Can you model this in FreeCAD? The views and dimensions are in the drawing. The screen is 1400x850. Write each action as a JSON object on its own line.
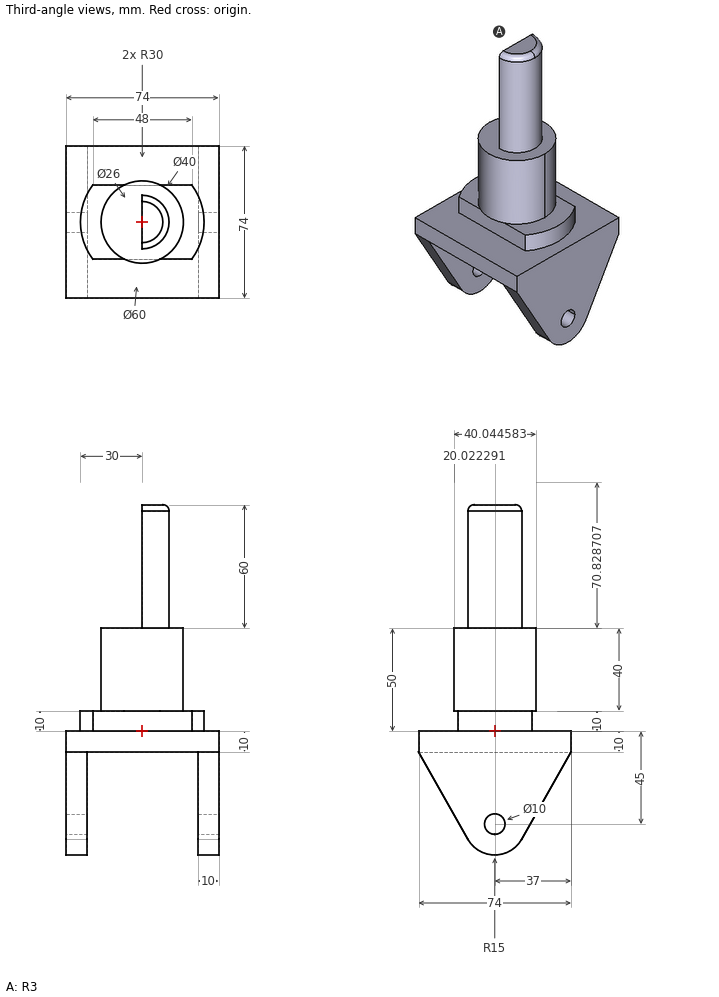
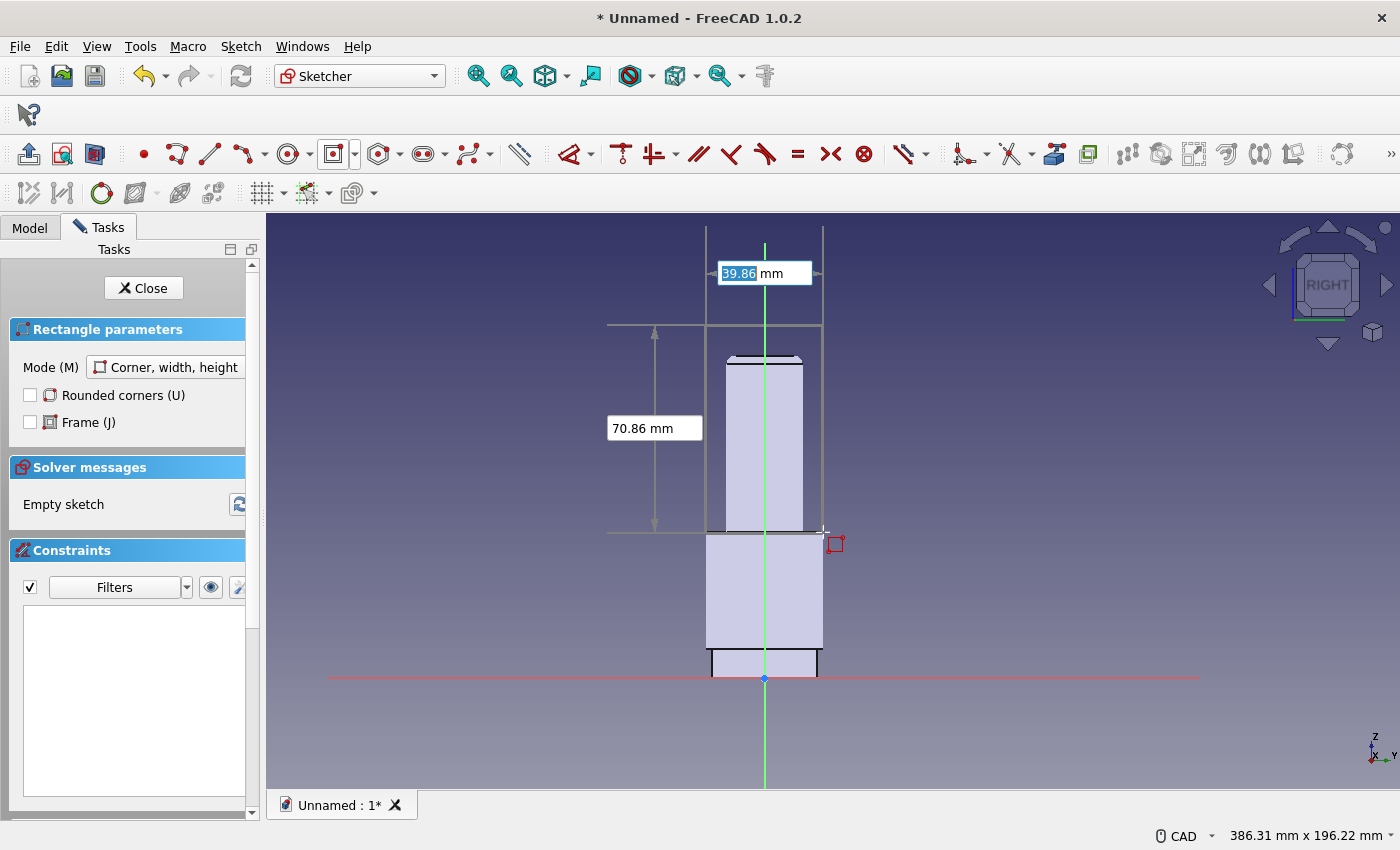
{"action": "type", "text": "40.044583"}
{"action": "key", "text": "Tab"}
{"action": "type", "text": "70.828707"}
{"action": "key", "text": "Return"}
{"action": "key", "text": "Escape"}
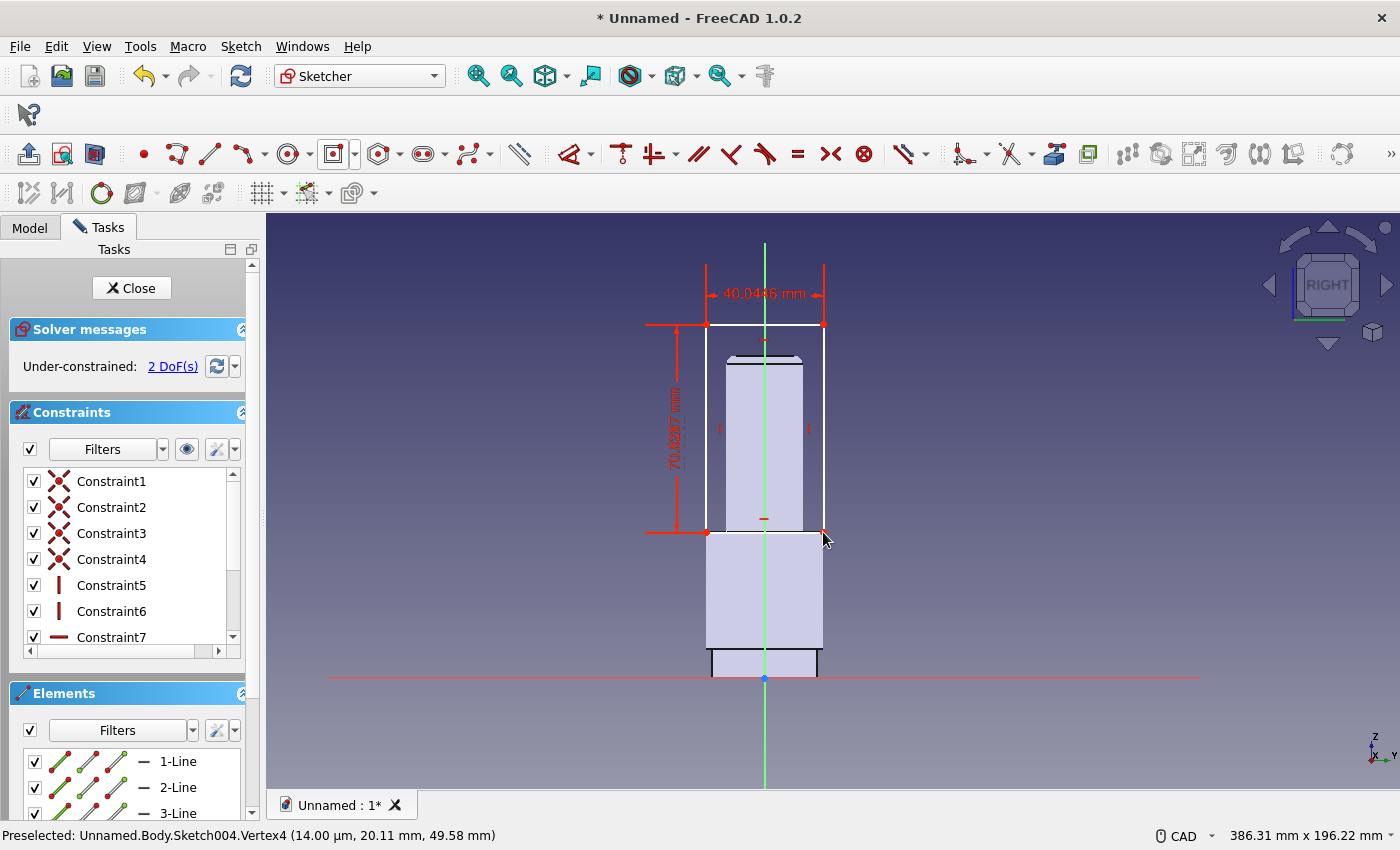
{"action": "left_click", "coordinate": [568, 154]}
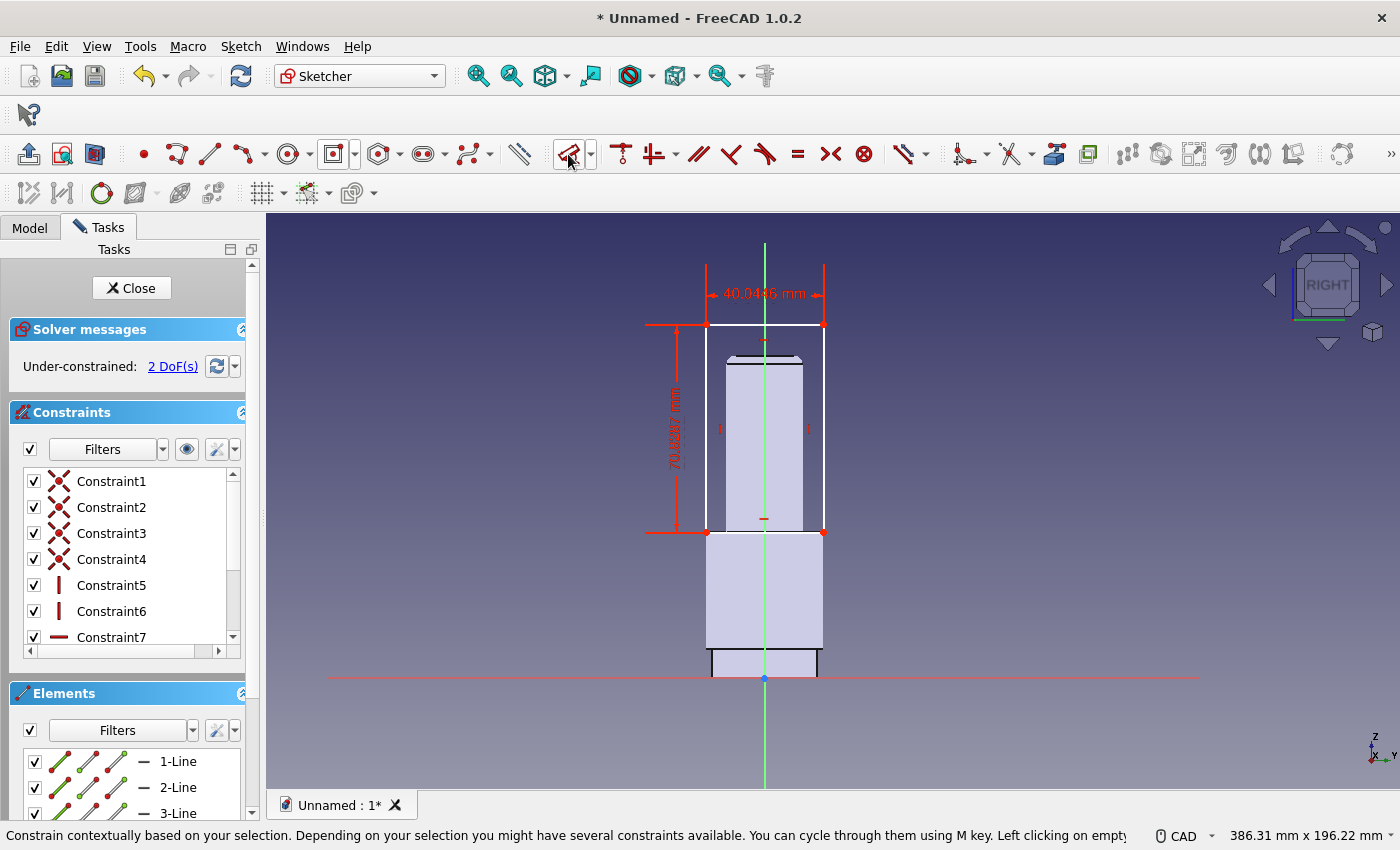
{"action": "left_click", "coordinate": [706, 533]}
{"action": "left_click", "coordinate": [672, 606]}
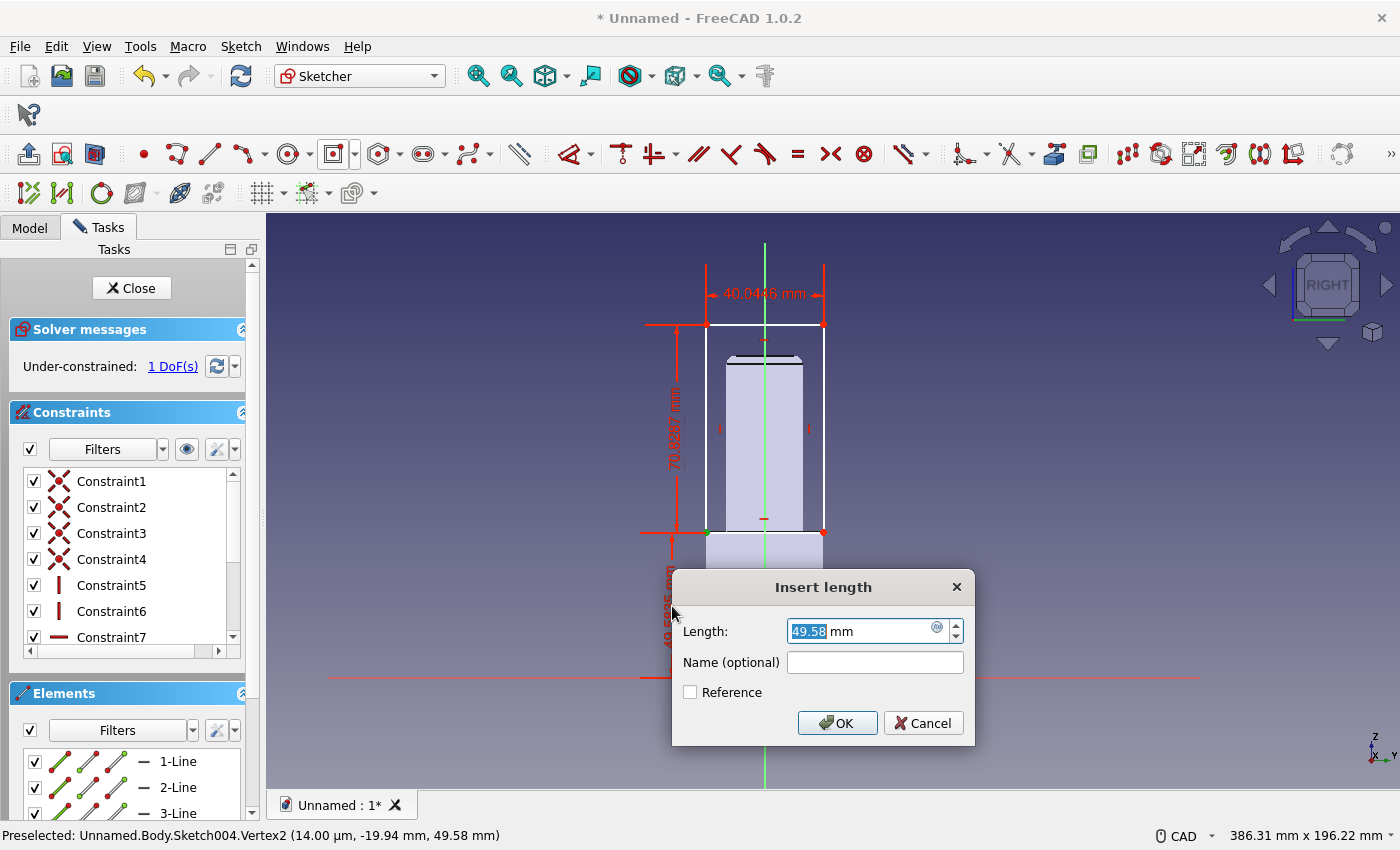
{"action": "type", "text": "50"}
{"action": "key", "text": "Return"}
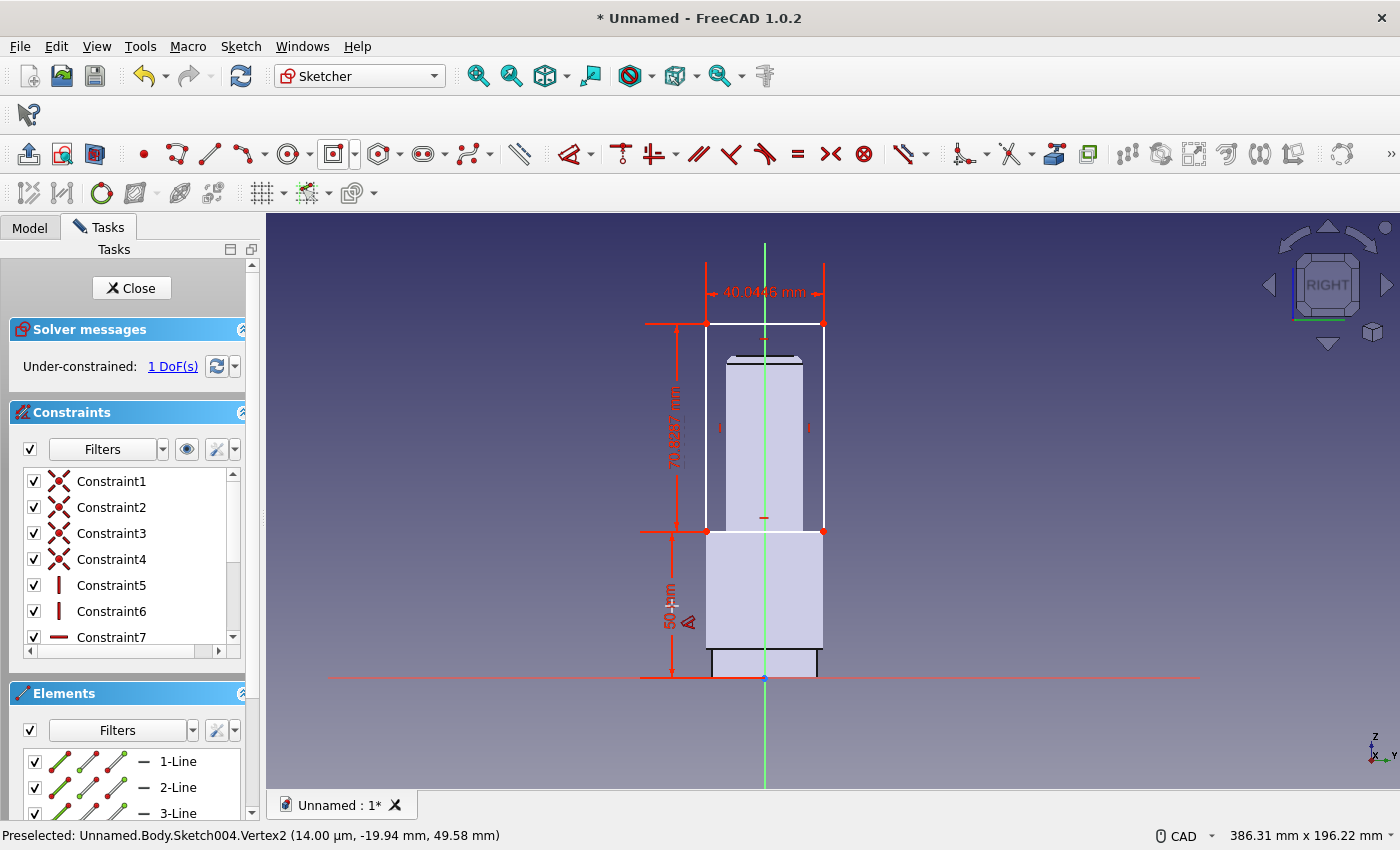
{"action": "left_click", "coordinate": [706, 324]}
{"action": "left_click", "coordinate": [735, 290]}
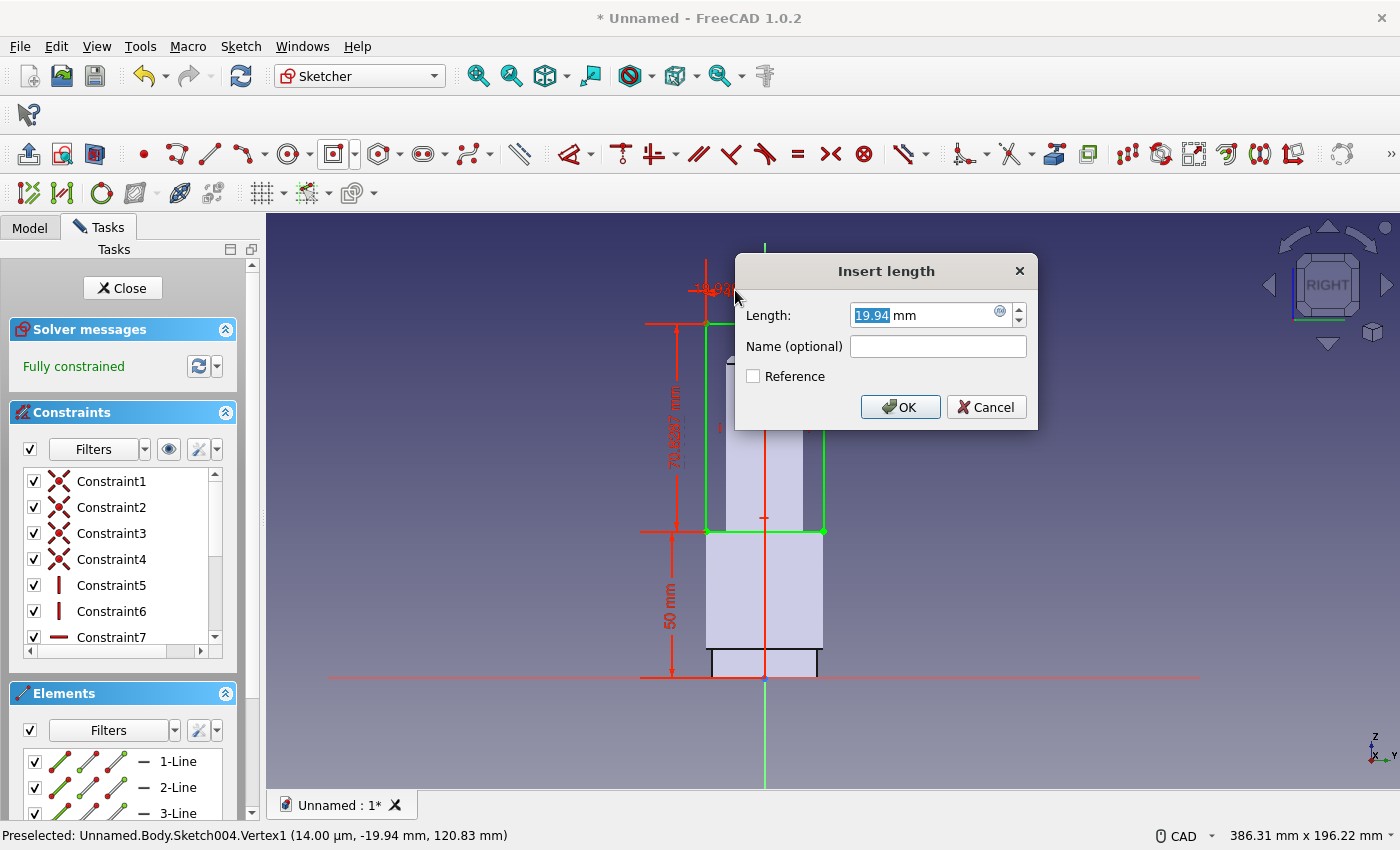
{"action": "type", "text": "20.022291"}
{"action": "key", "text": "Return"}
{"action": "key", "text": "Escape"}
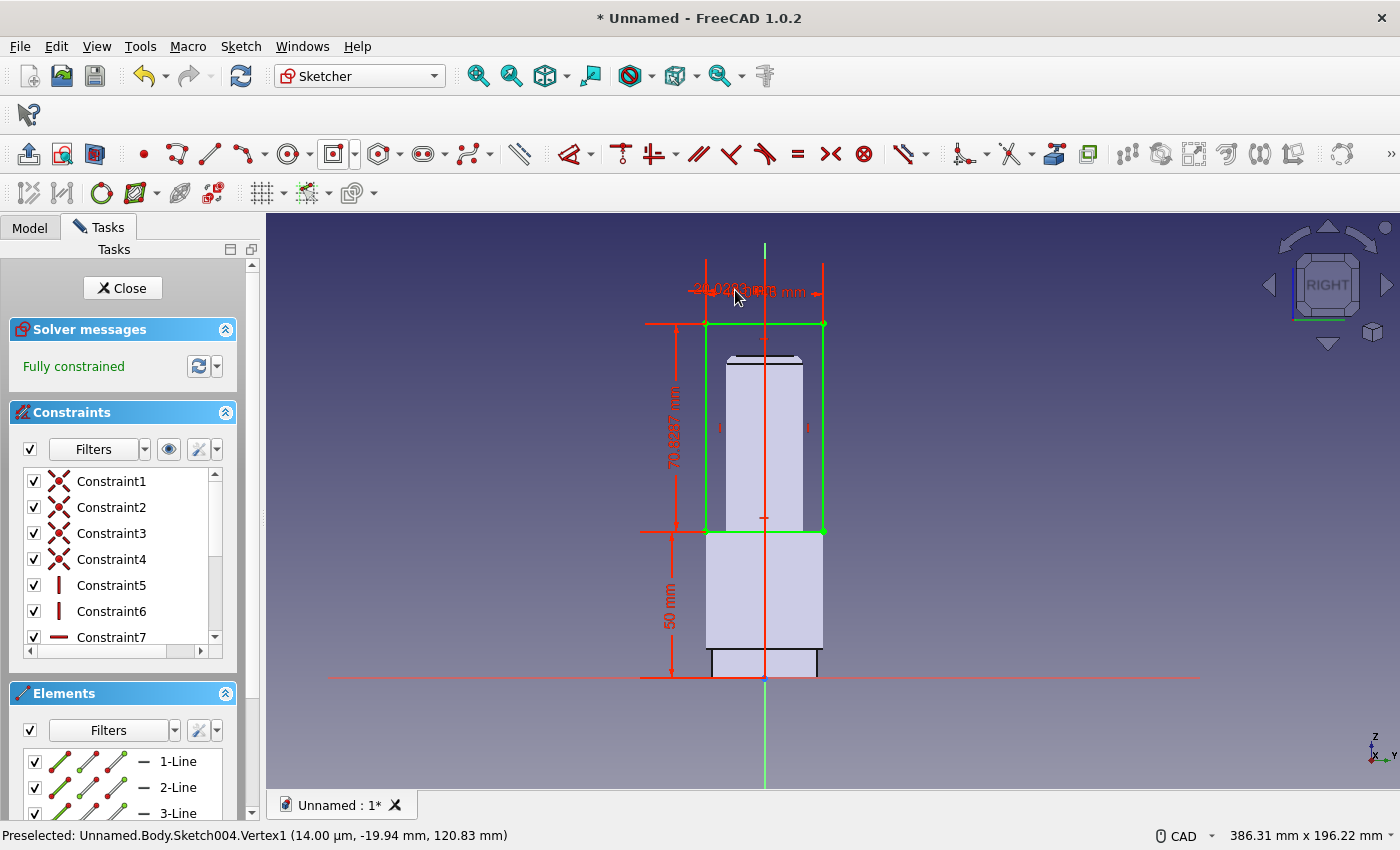
{"action": "left_click", "coordinate": [123, 288]}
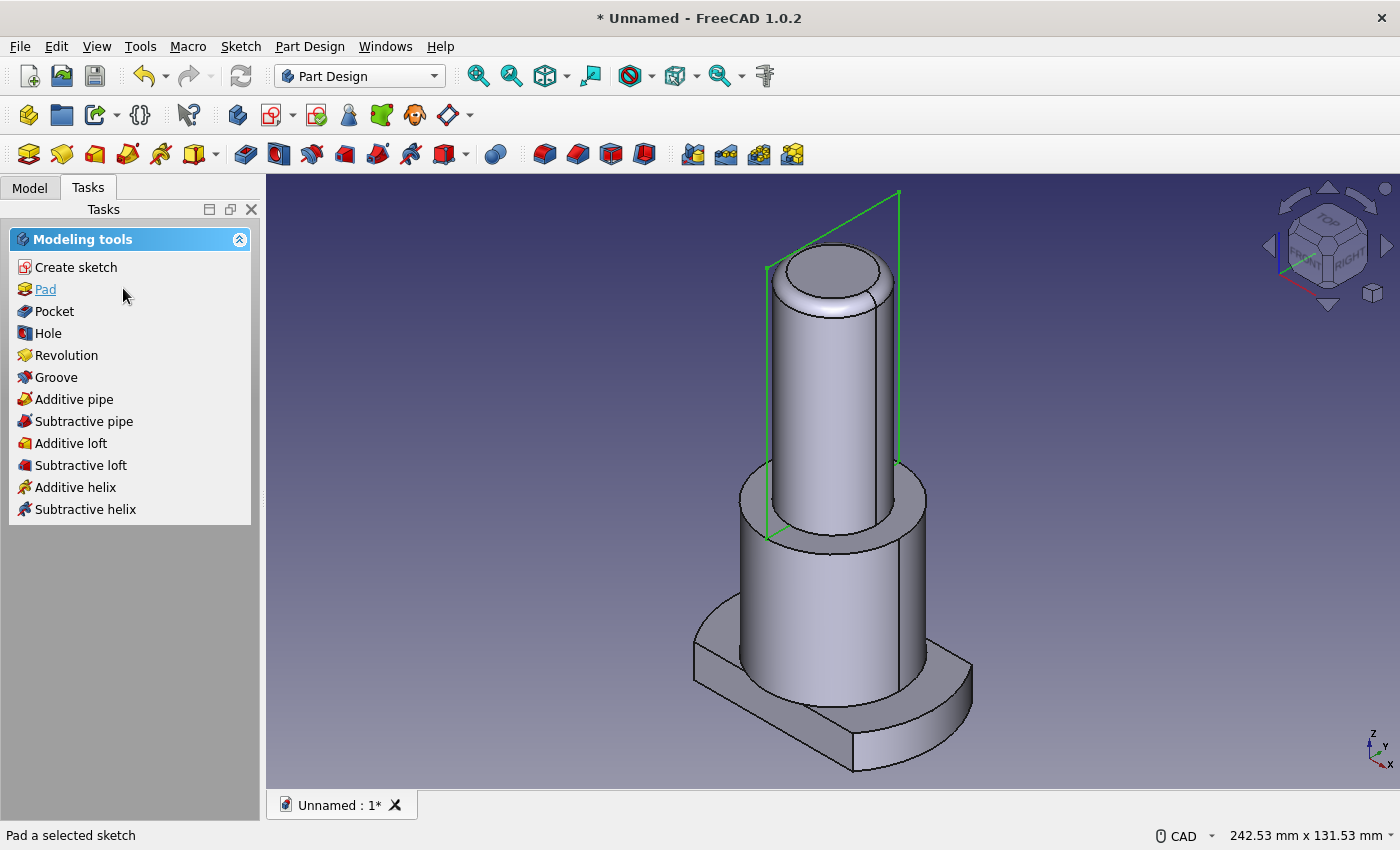
{"action": "left_click", "coordinate": [246, 154]}